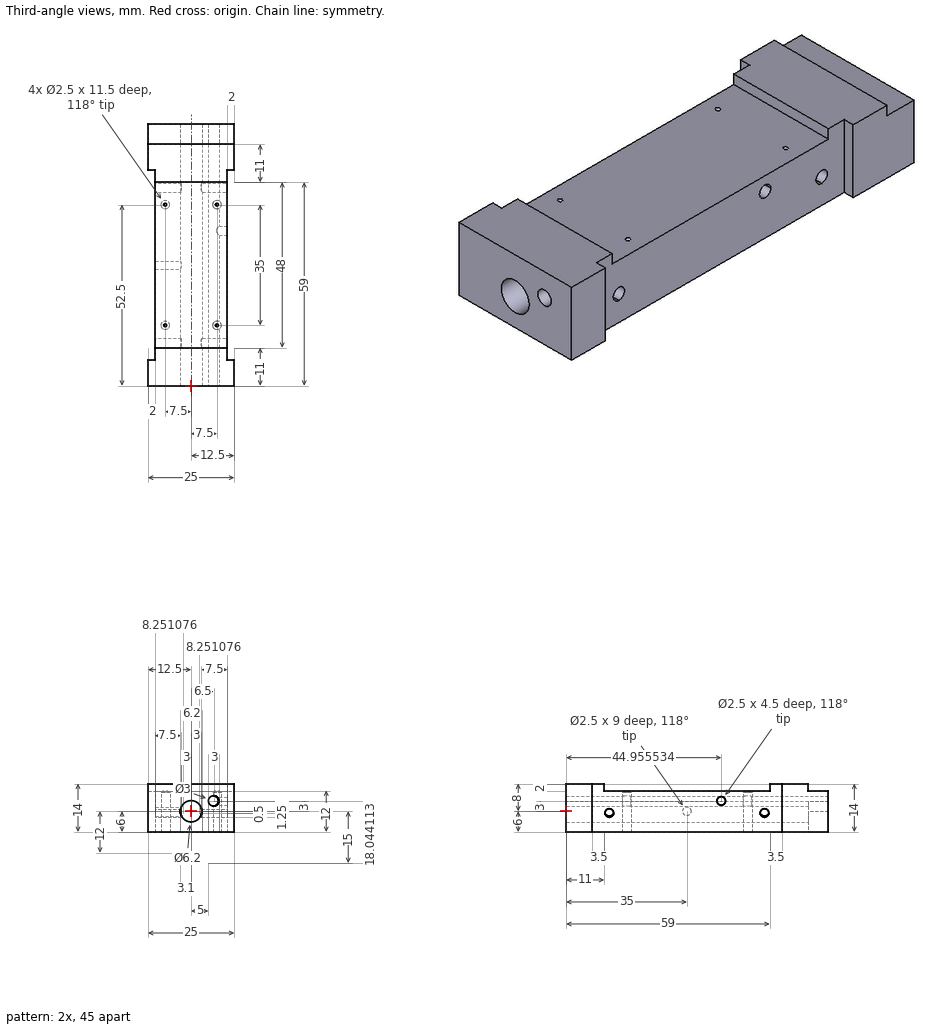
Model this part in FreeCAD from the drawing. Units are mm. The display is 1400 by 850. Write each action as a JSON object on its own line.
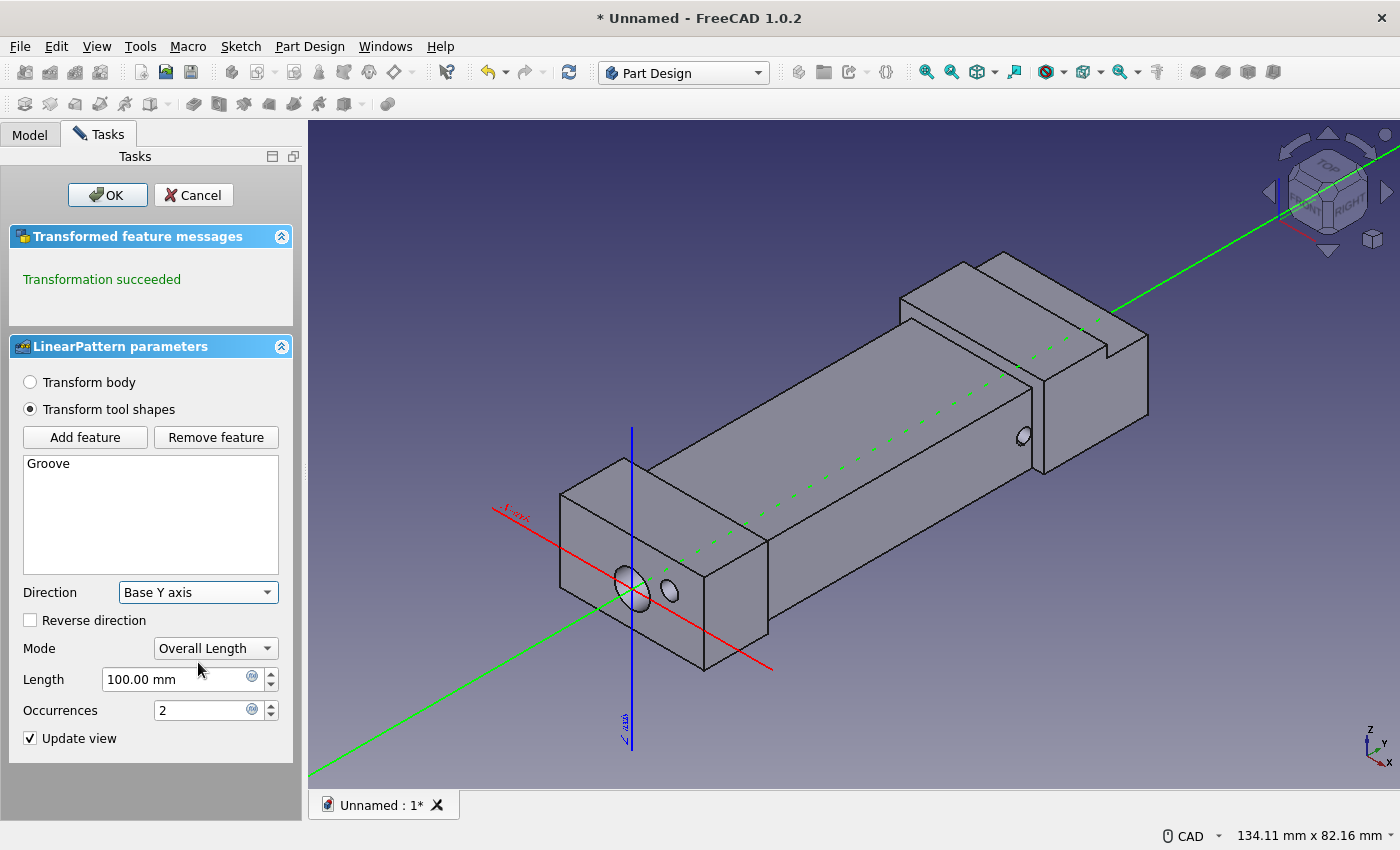
{"action": "left_click", "coordinate": [216, 648]}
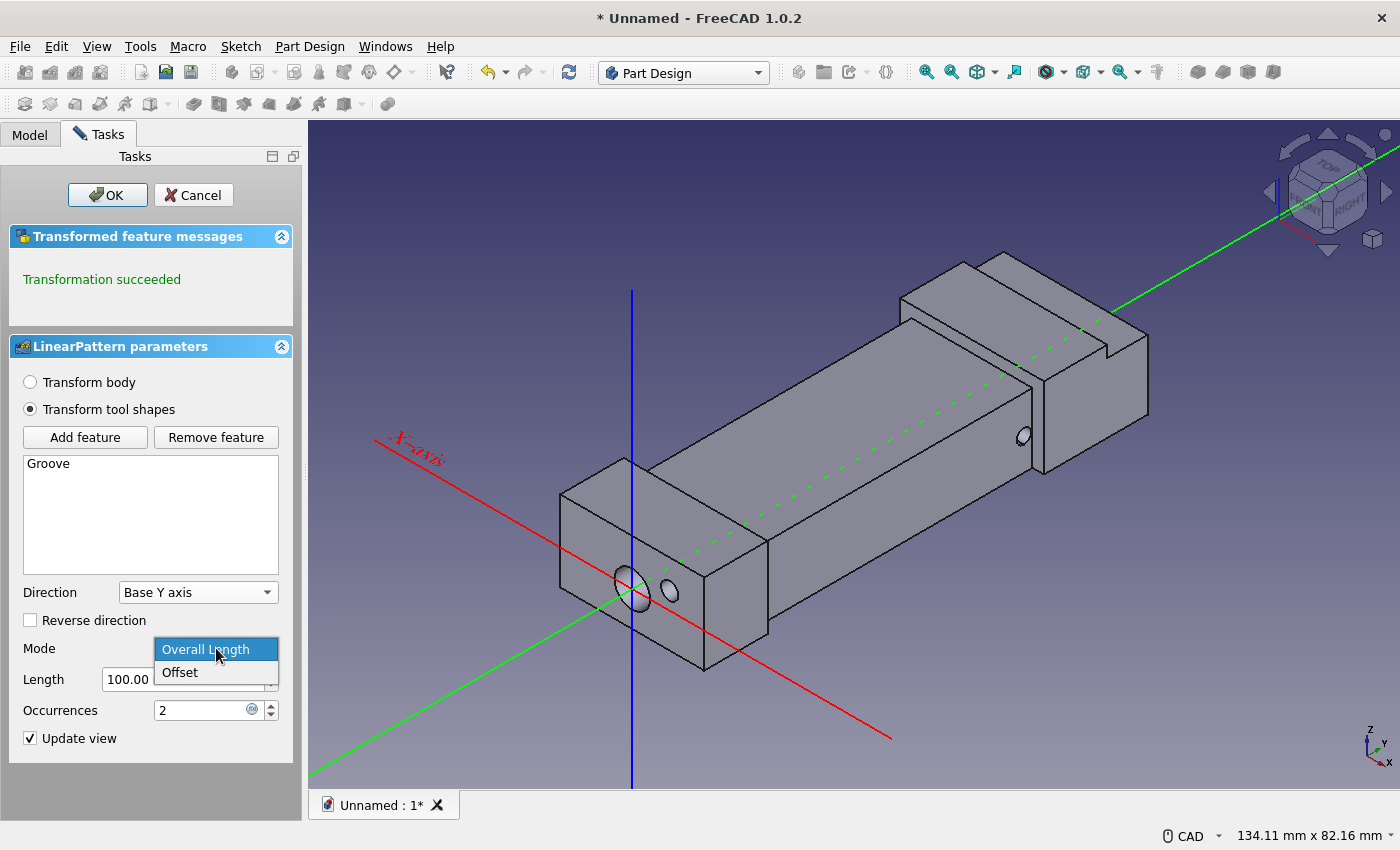
{"action": "left_click", "coordinate": [214, 672]}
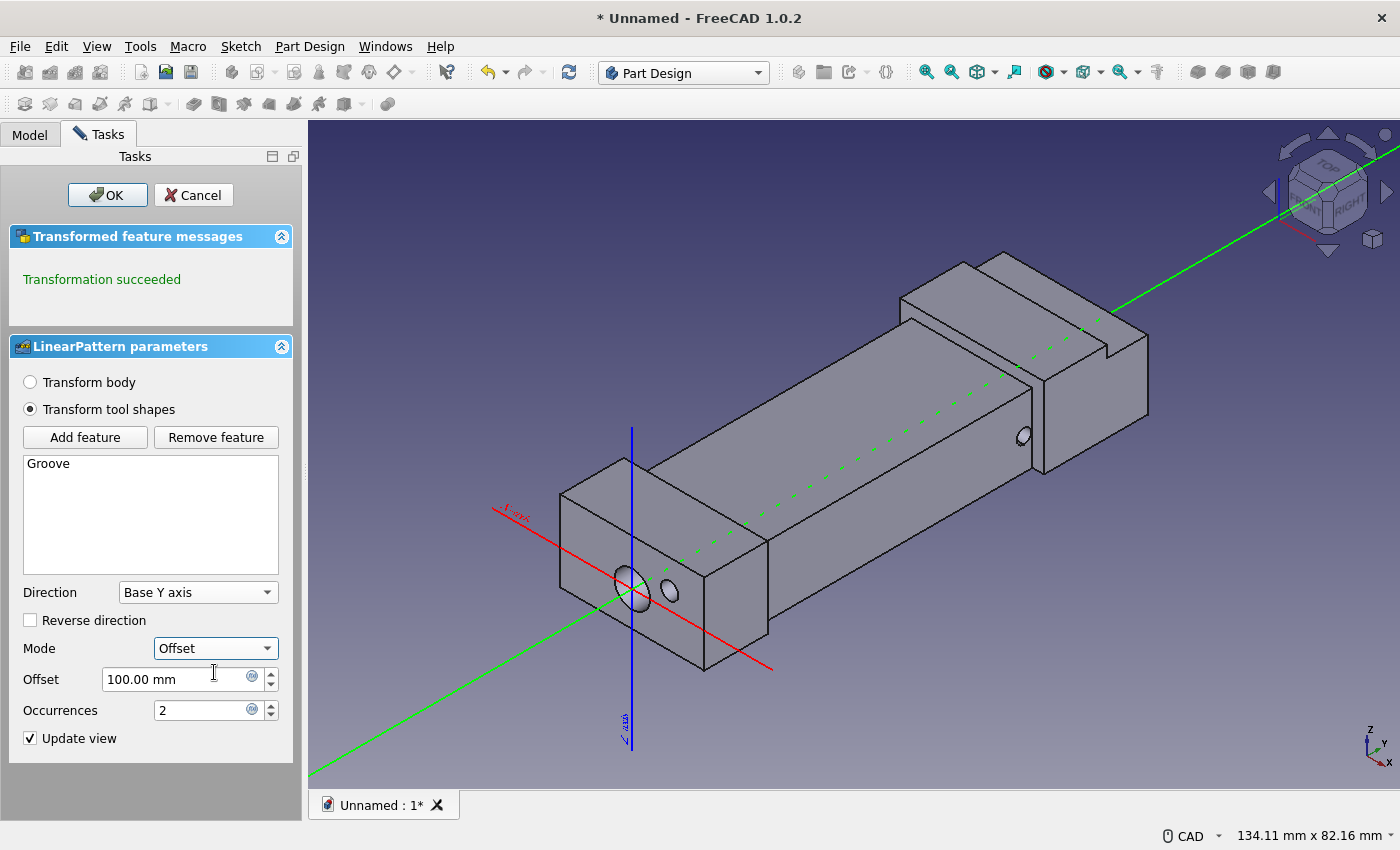
{"action": "triple_click", "coordinate": [184, 680]}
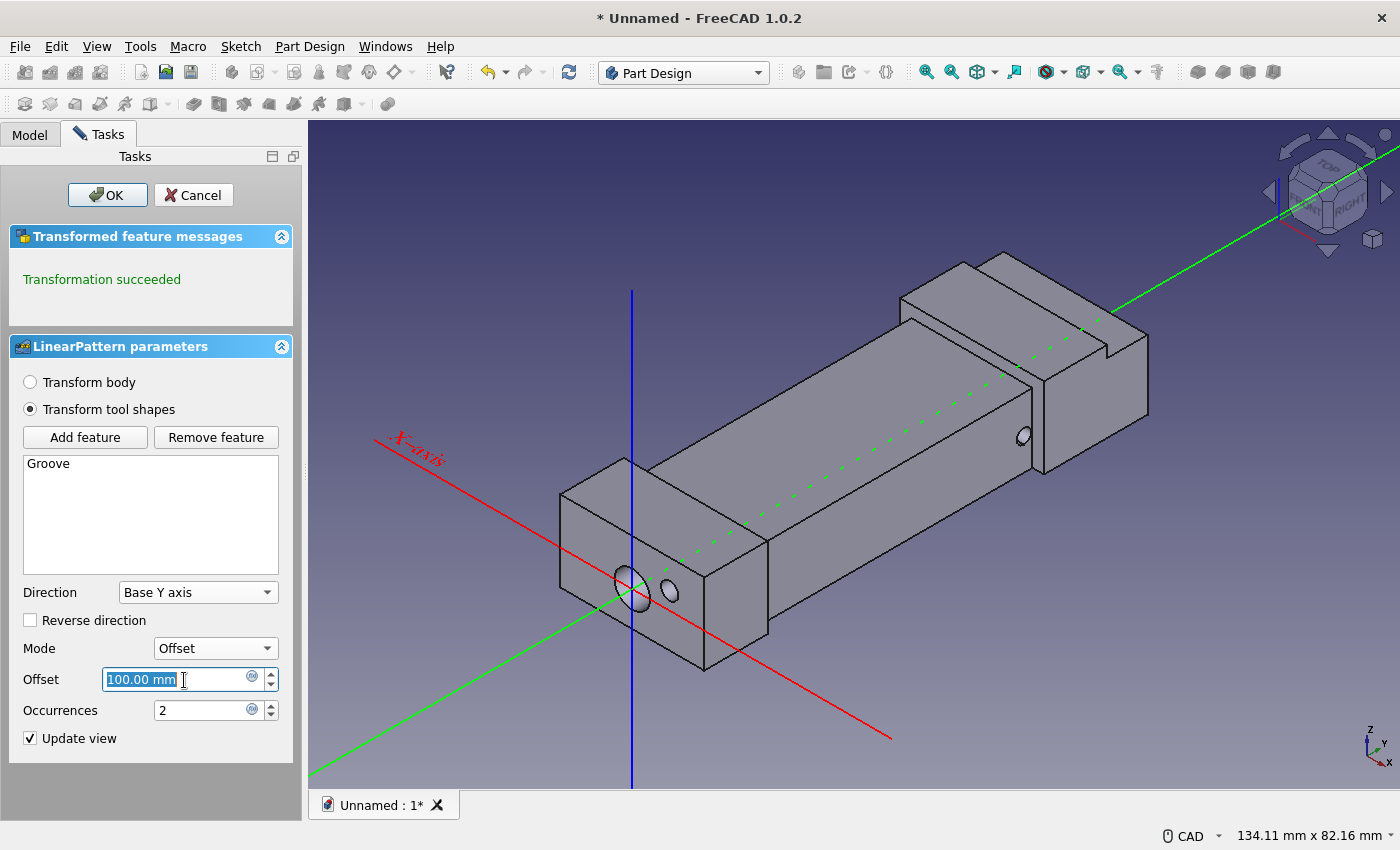
{"action": "type", "text": "45"}
{"action": "key", "text": "Tab"}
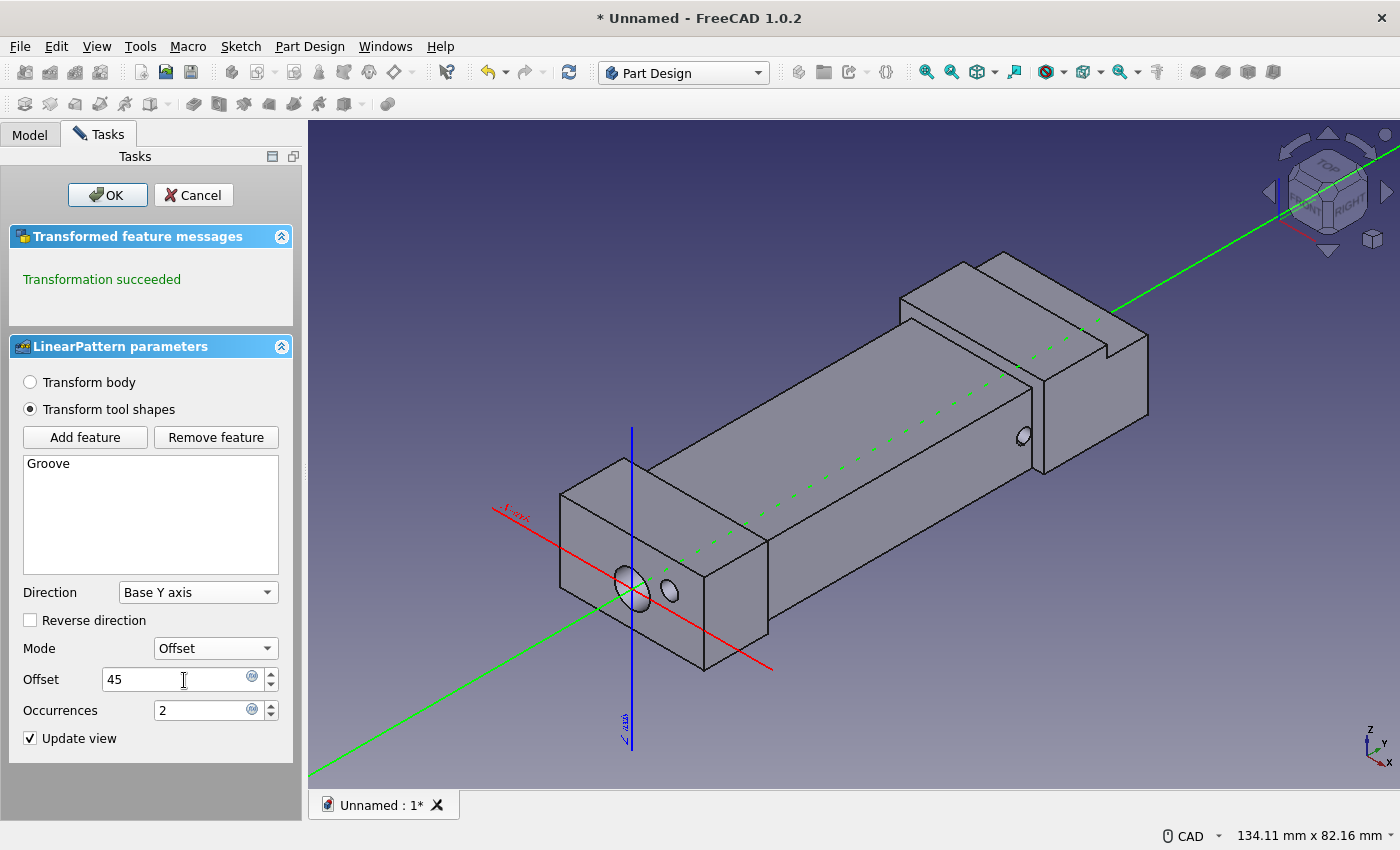
{"action": "triple_click", "coordinate": [210, 710]}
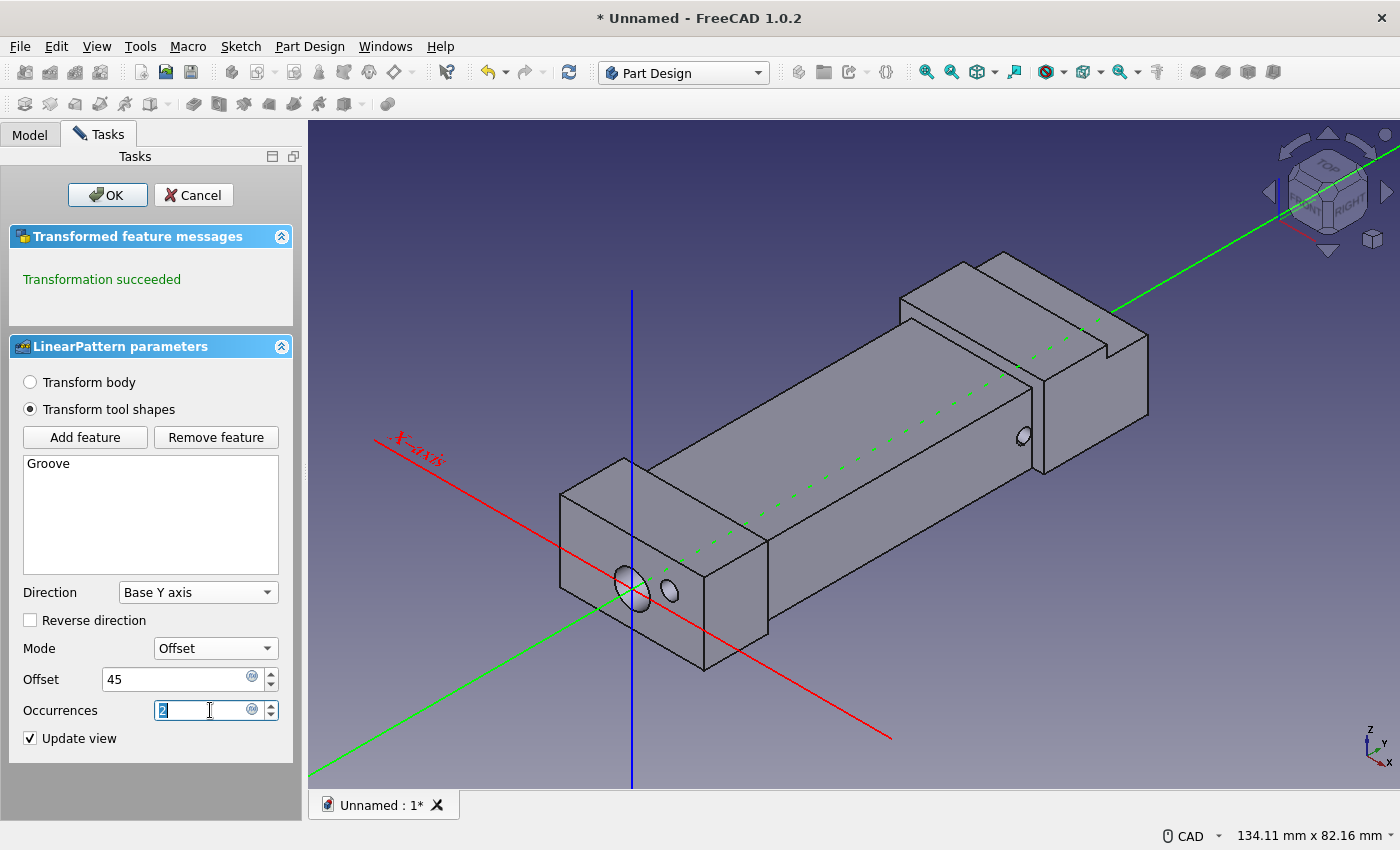
{"action": "type", "text": "2"}
{"action": "key", "text": "Tab"}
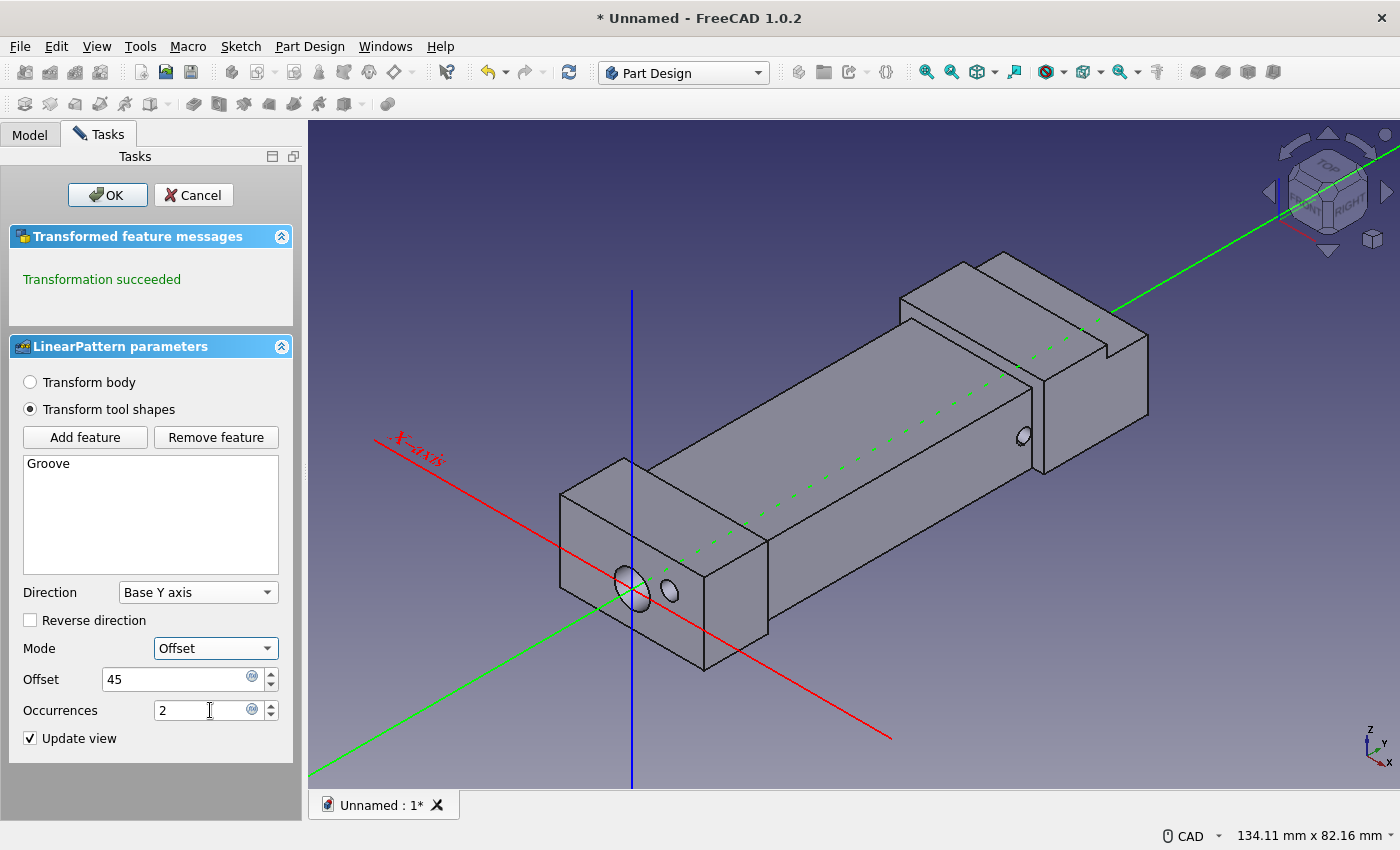
{"action": "left_click", "coordinate": [31, 620]}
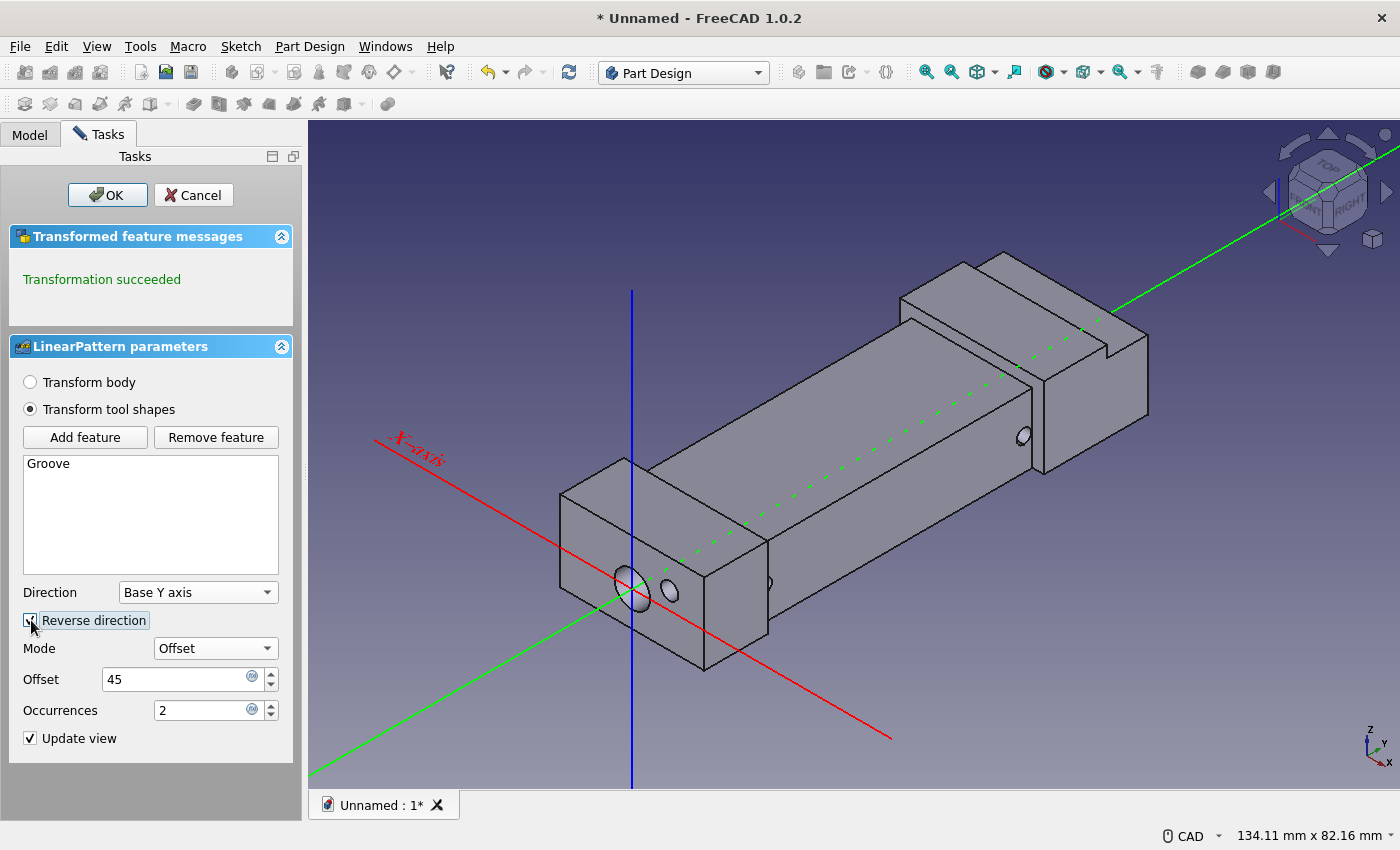
{"action": "left_click", "coordinate": [108, 195]}